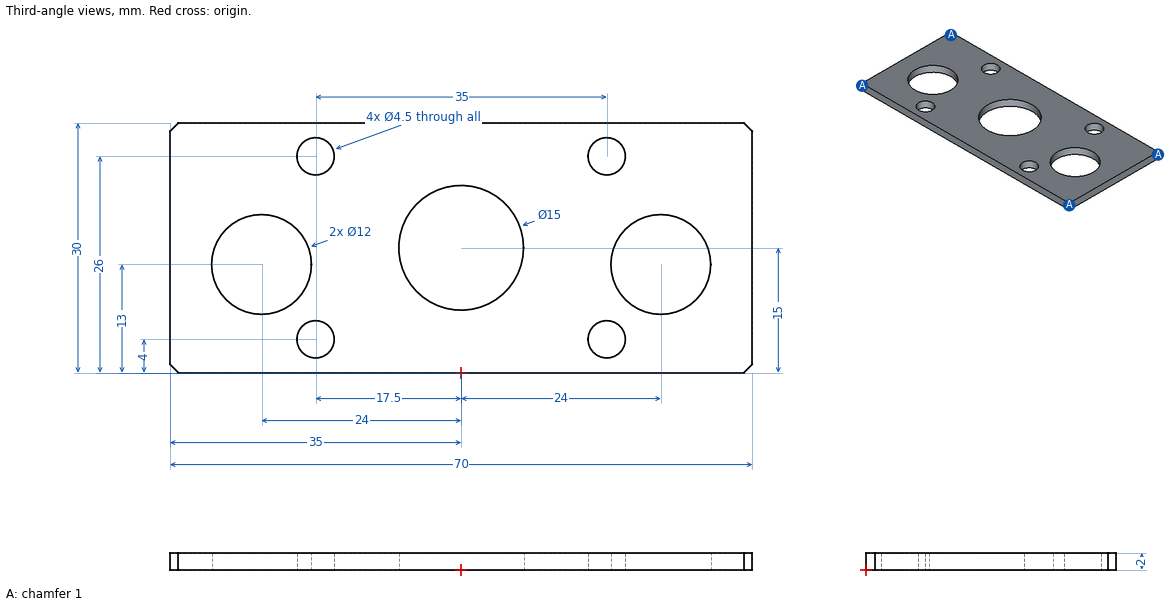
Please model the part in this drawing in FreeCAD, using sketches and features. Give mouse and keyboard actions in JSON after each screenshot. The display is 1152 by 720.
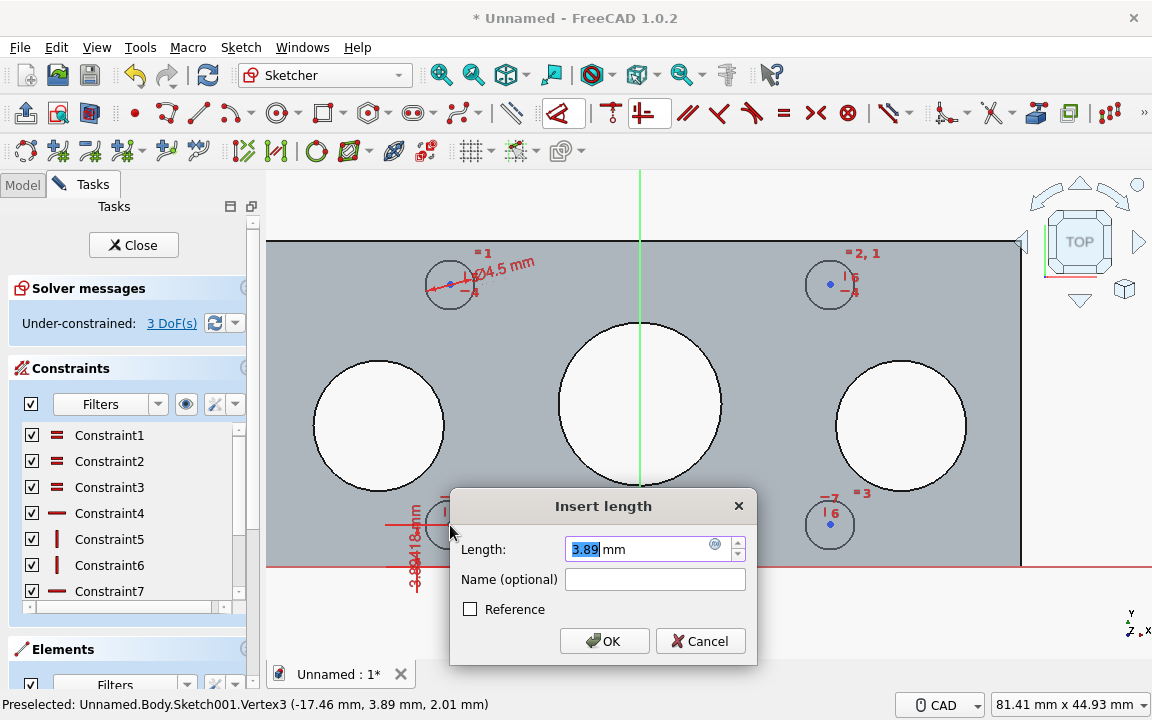
{"action": "type", "text": "4"}
{"action": "key", "text": "Return"}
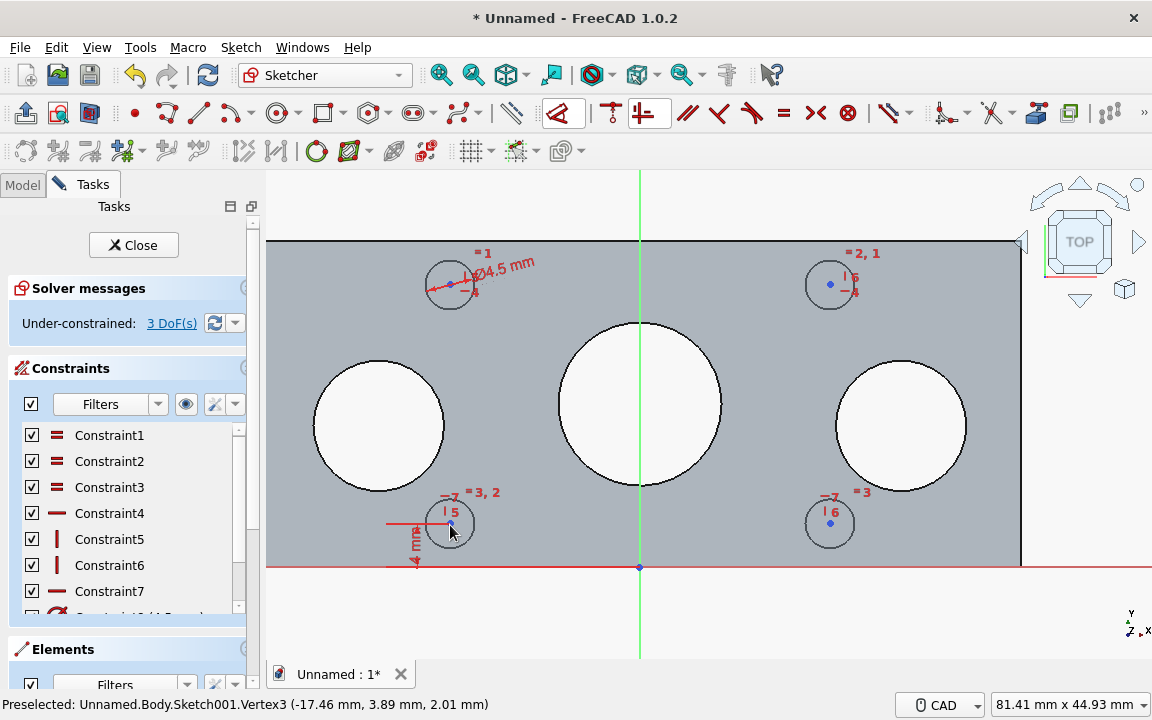
{"action": "left_click", "coordinate": [450, 285]}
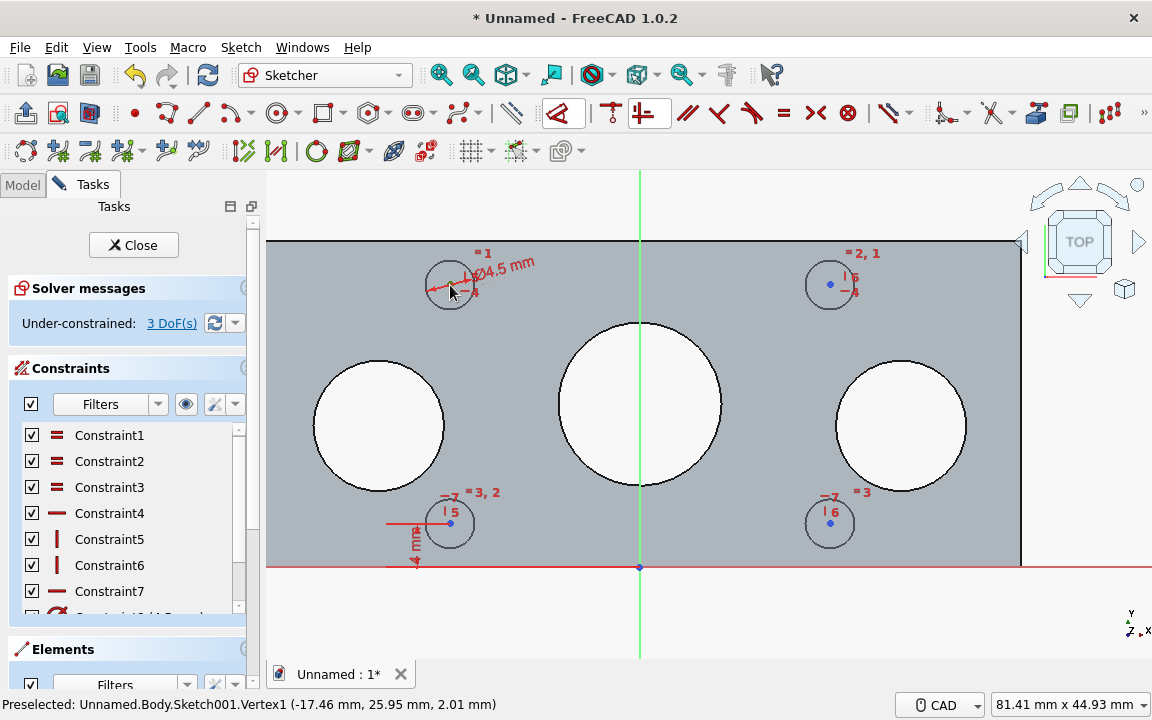
{"action": "left_click", "coordinate": [580, 114]}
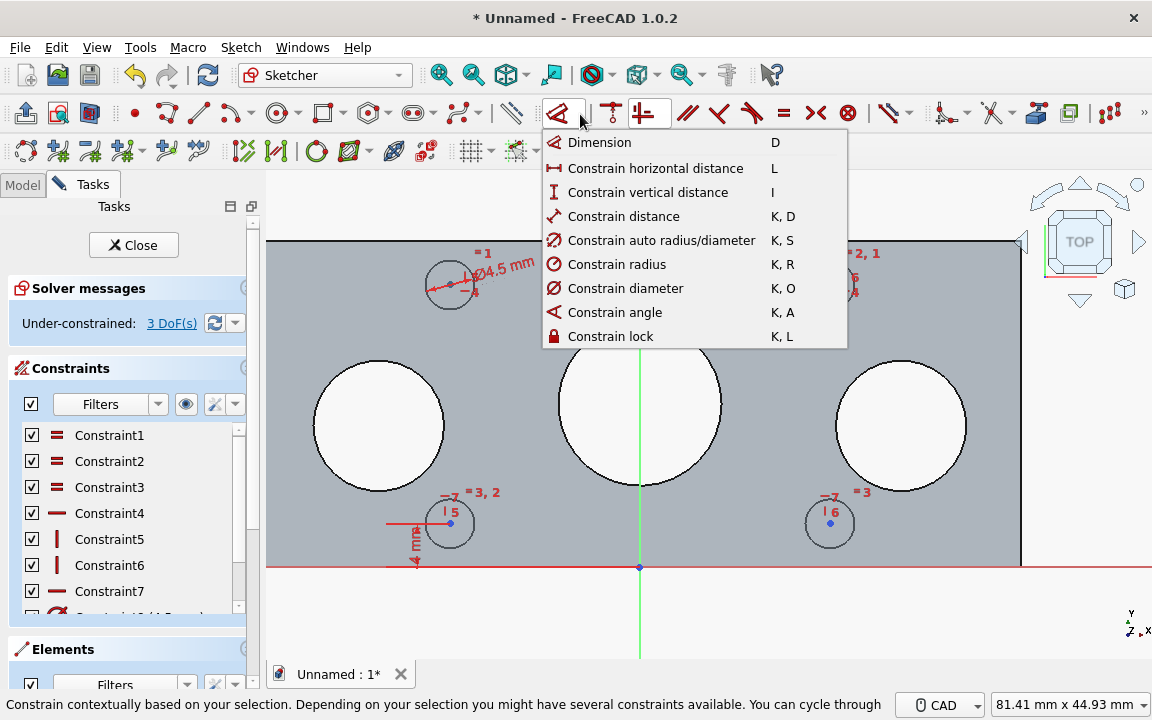
{"action": "left_click", "coordinate": [695, 192]}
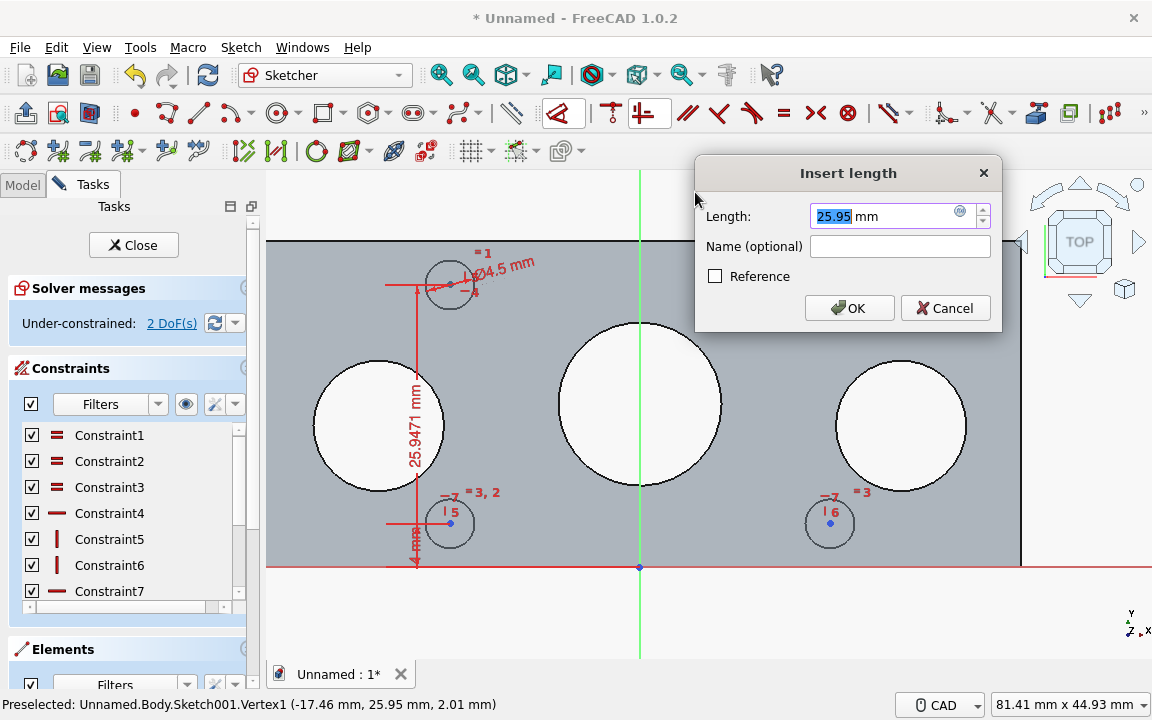
{"action": "type", "text": "26"}
{"action": "key", "text": "Return"}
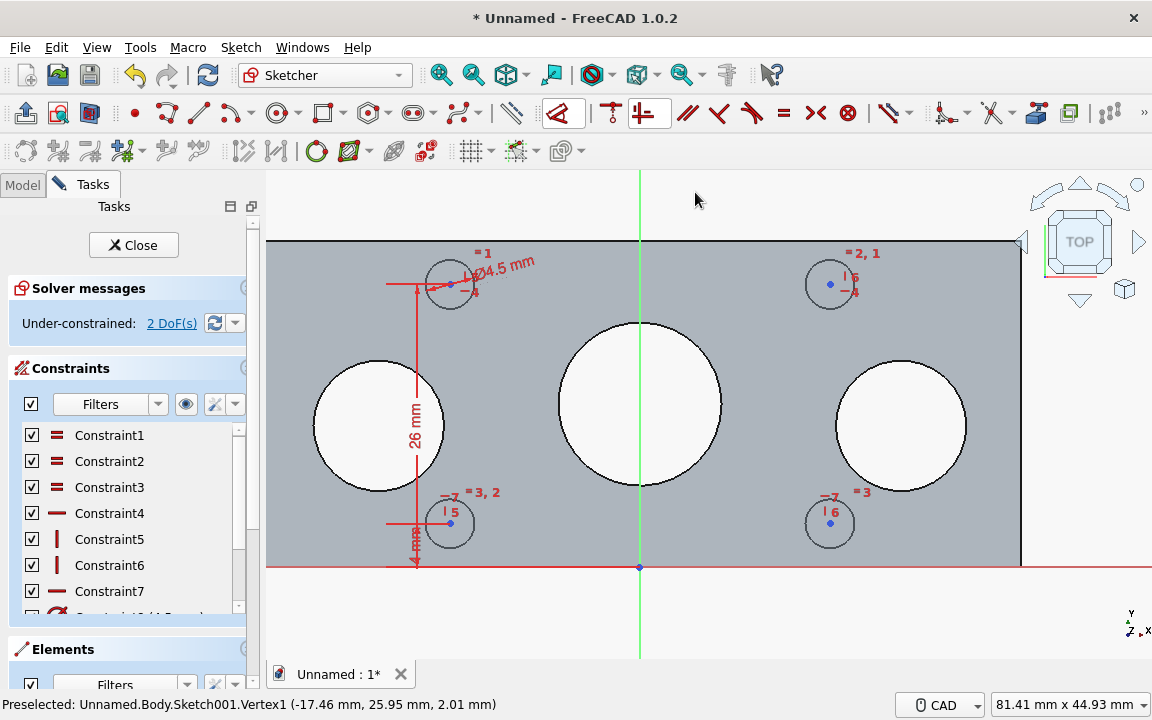
{"action": "left_click", "coordinate": [450, 284]}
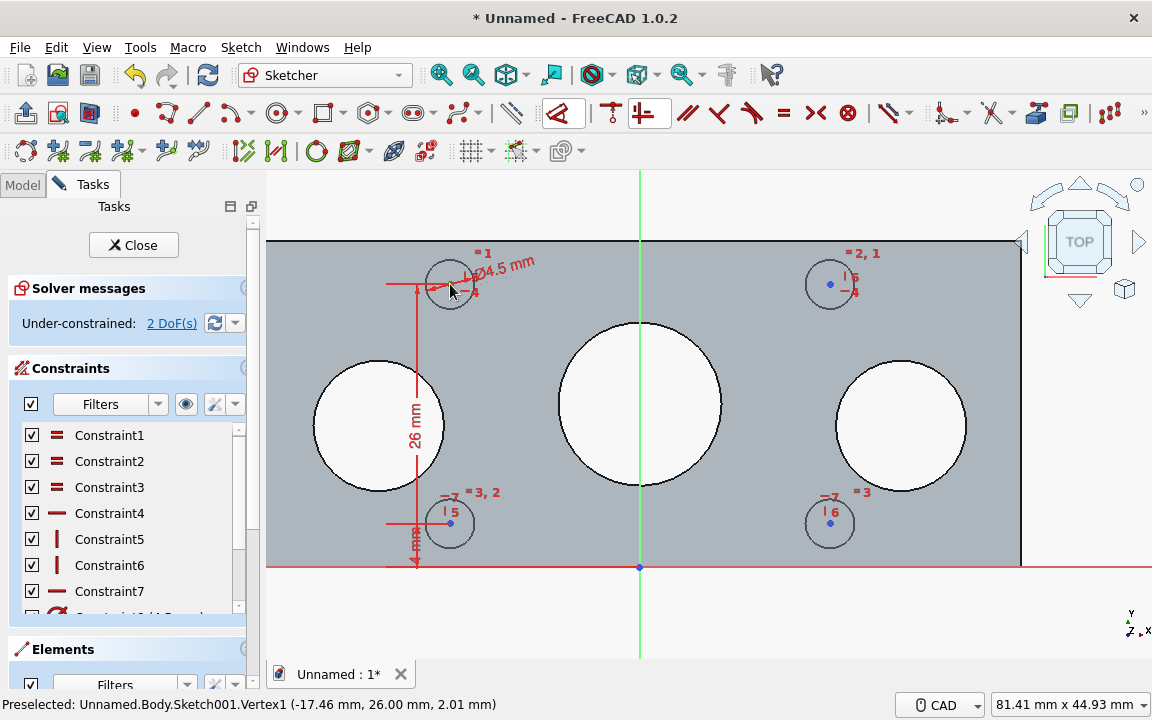
{"action": "left_click", "coordinate": [830, 284]}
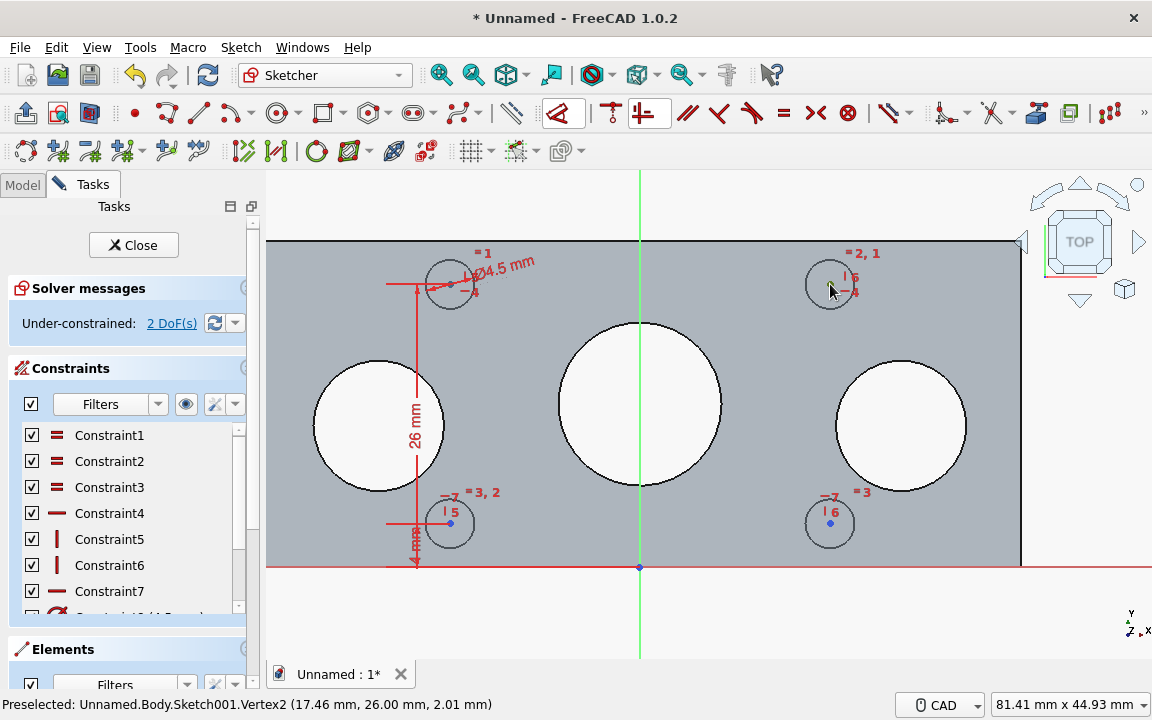
{"action": "key", "text": "l"}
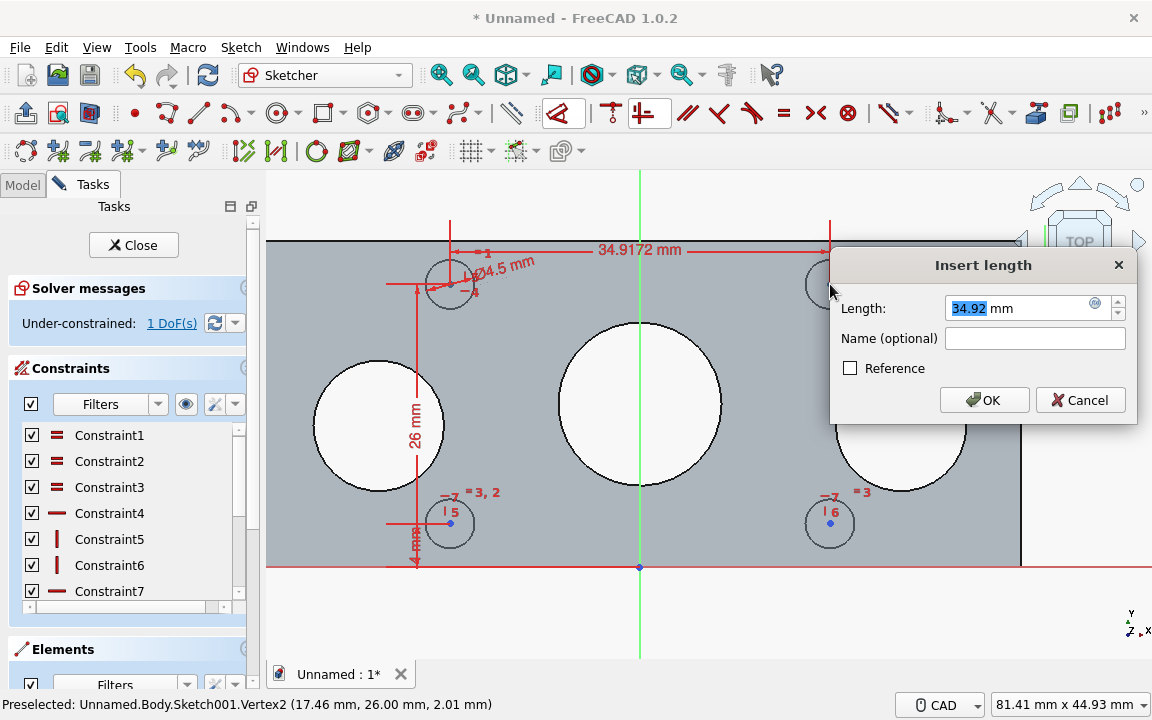
{"action": "type", "text": "35"}
{"action": "key", "text": "Return"}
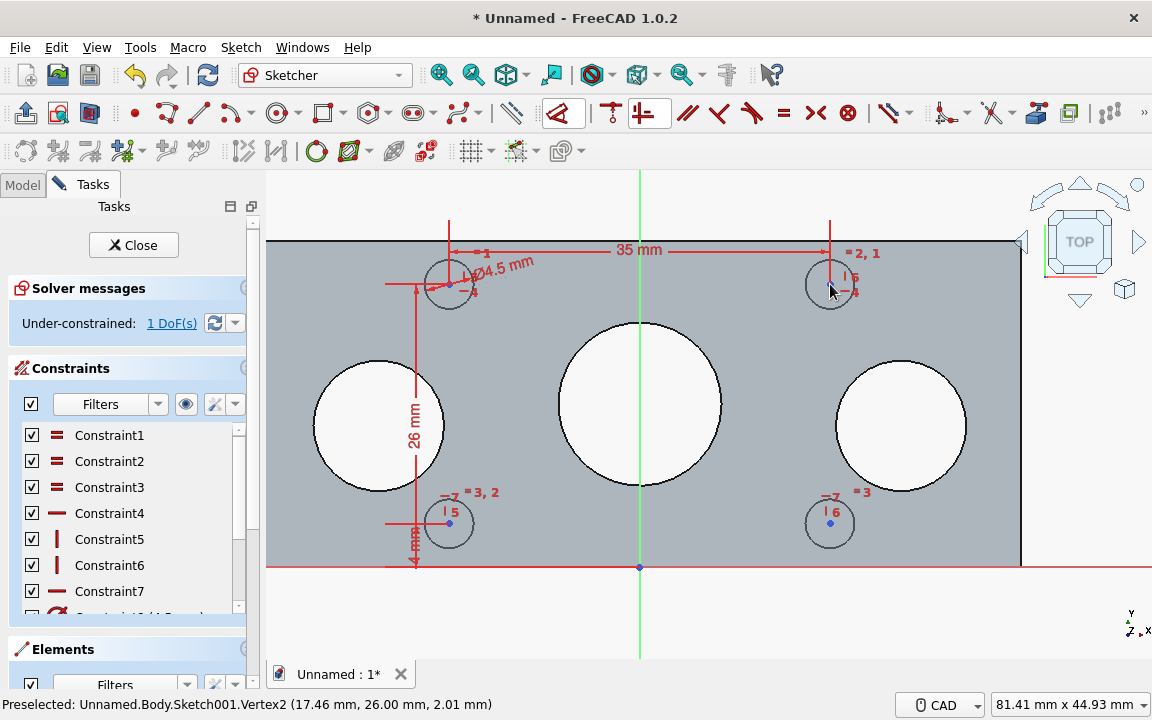
{"action": "left_click", "coordinate": [449, 284]}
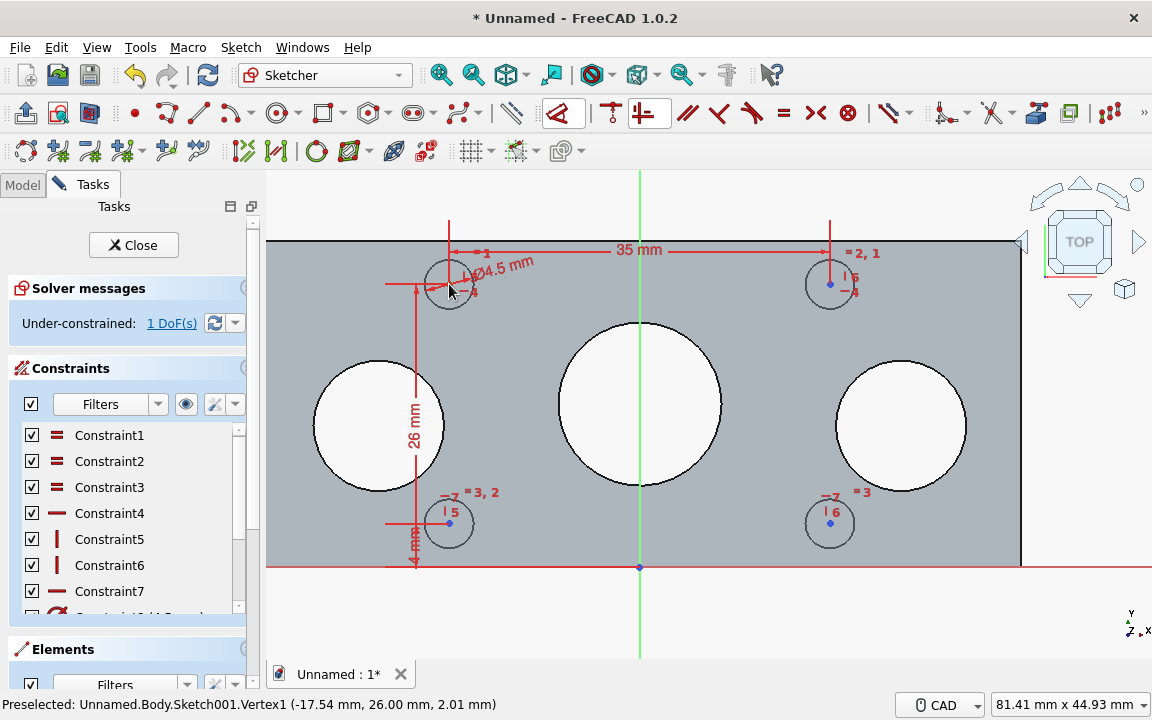
{"action": "left_click", "coordinate": [580, 114]}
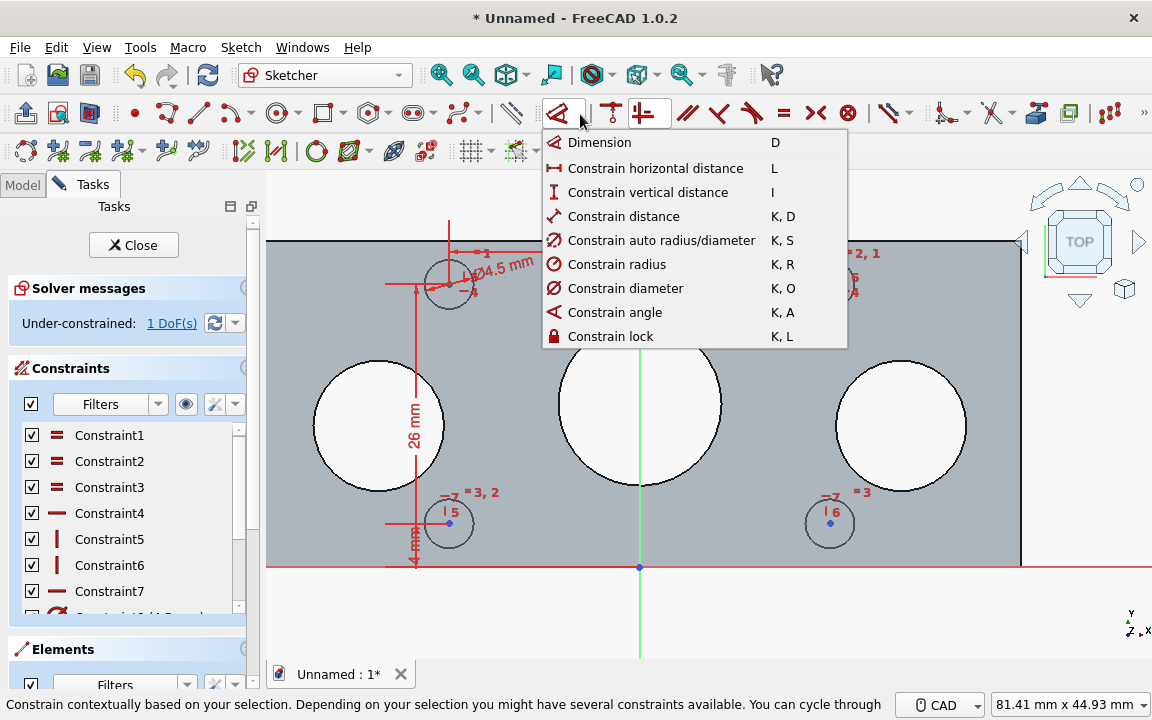
{"action": "left_click", "coordinate": [695, 168]}